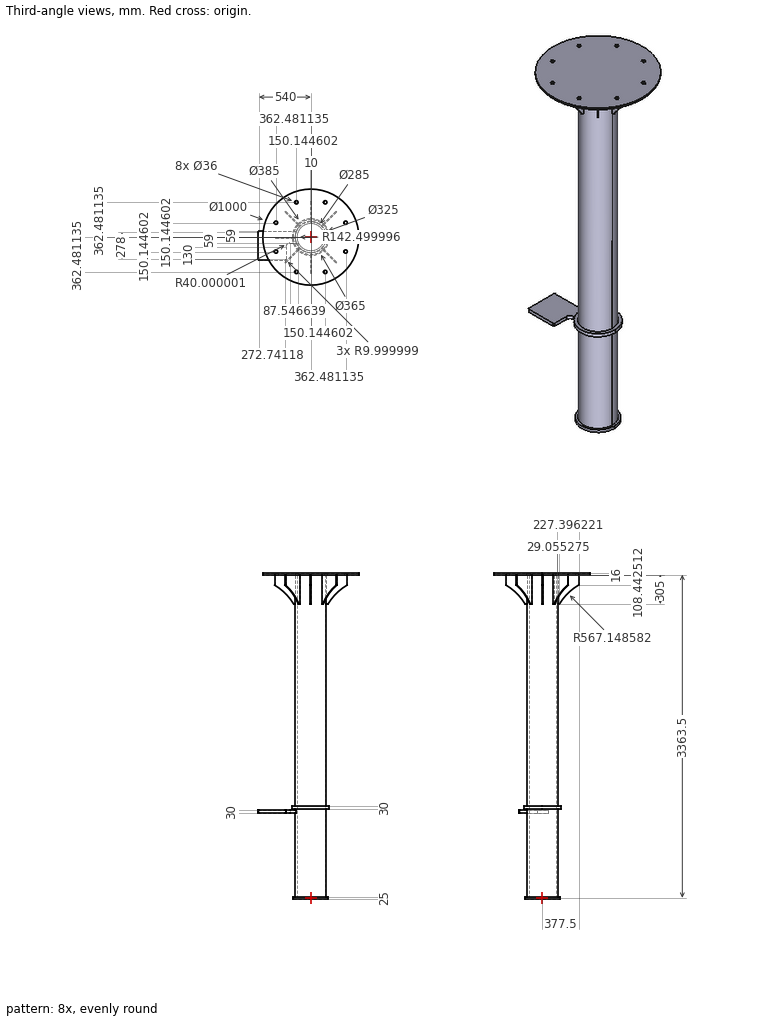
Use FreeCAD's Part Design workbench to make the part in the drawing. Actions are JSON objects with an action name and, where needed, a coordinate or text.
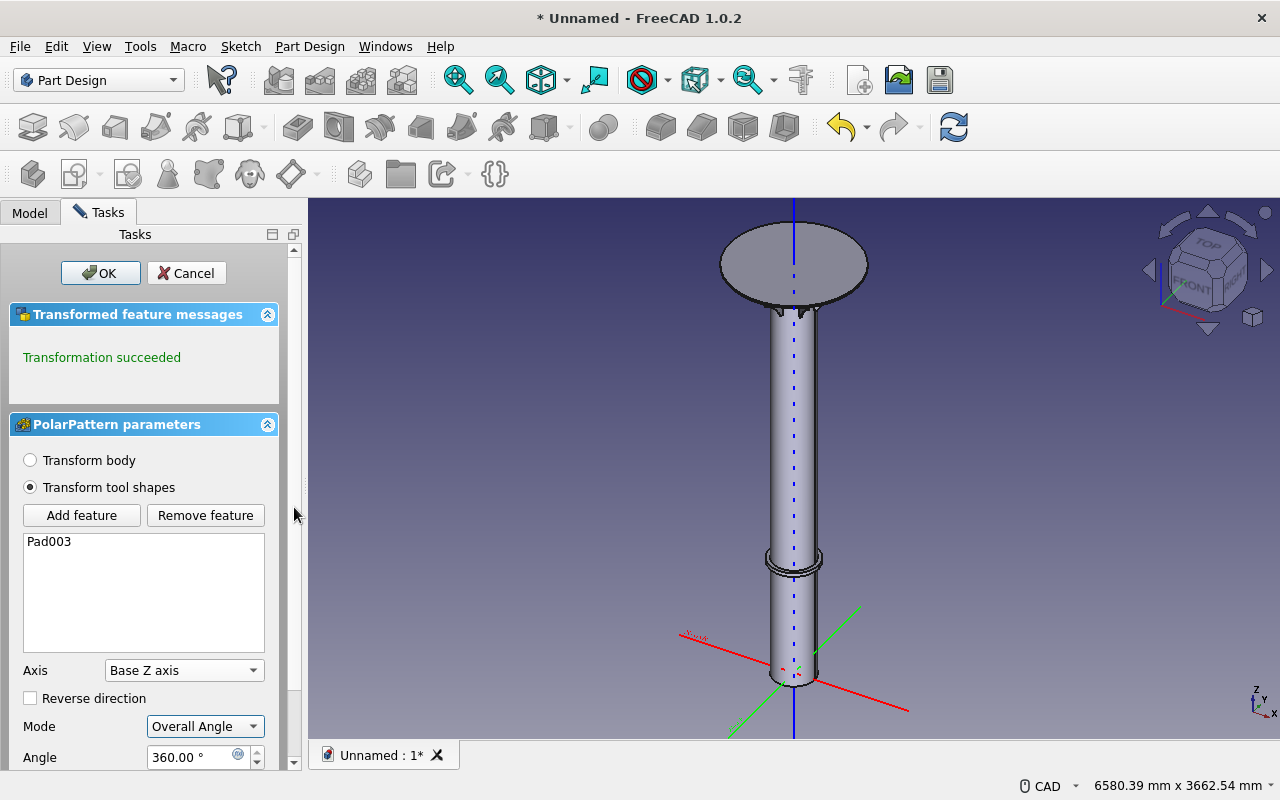
{"action": "left_click", "coordinate": [101, 273]}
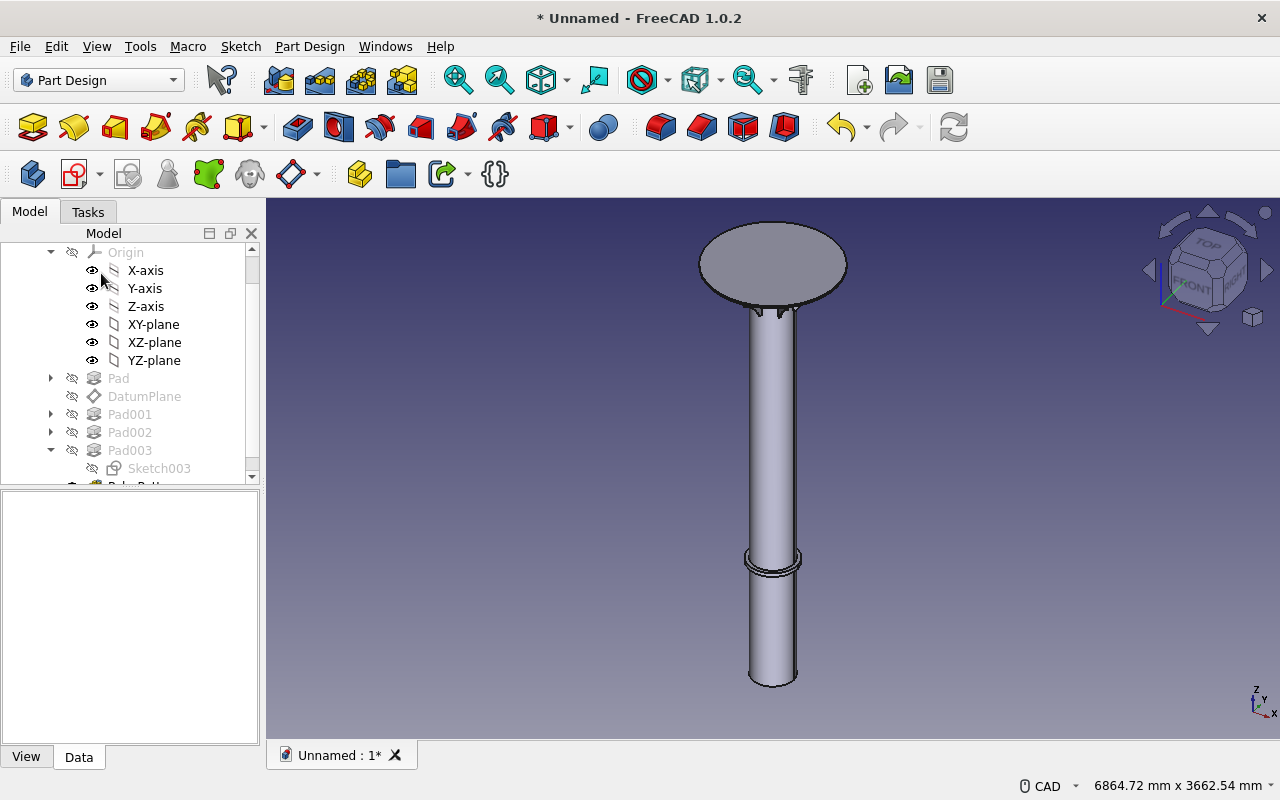
{"action": "key", "text": "5"}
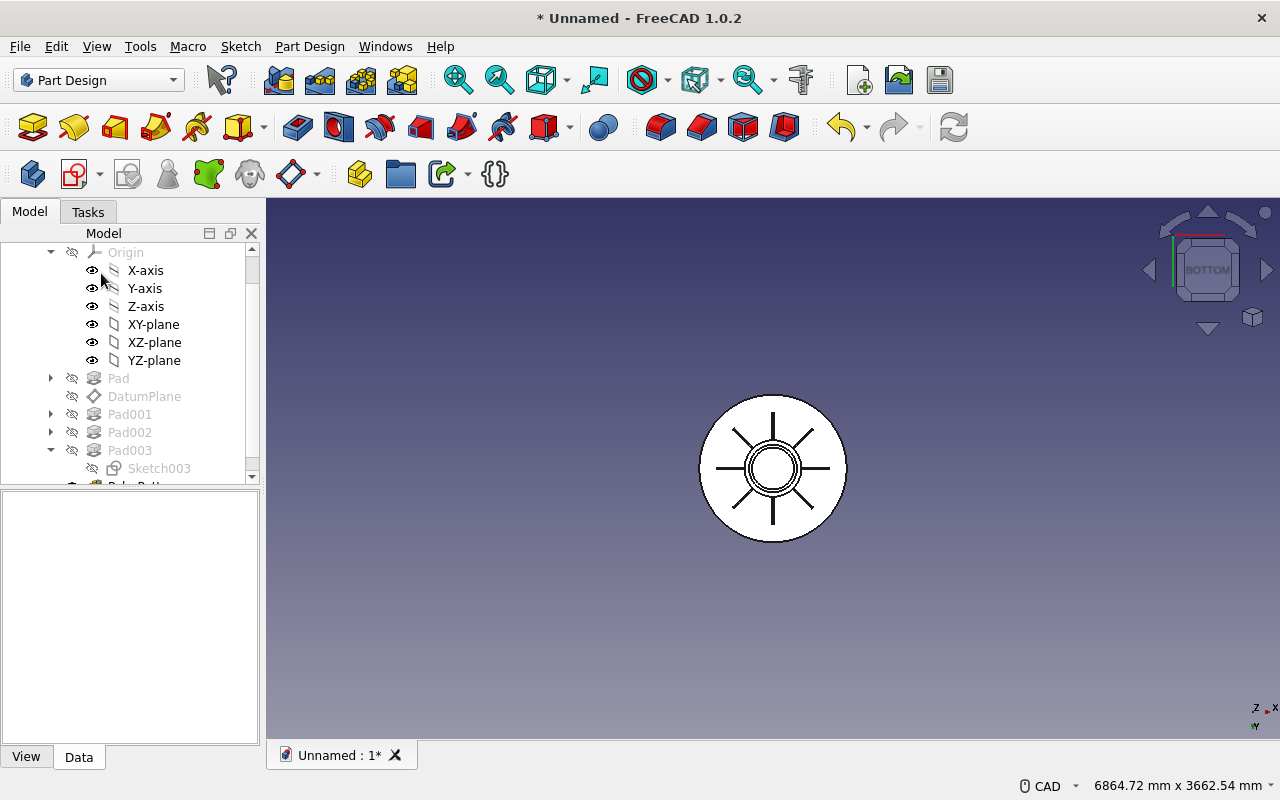
{"action": "left_click", "coordinate": [459, 80]}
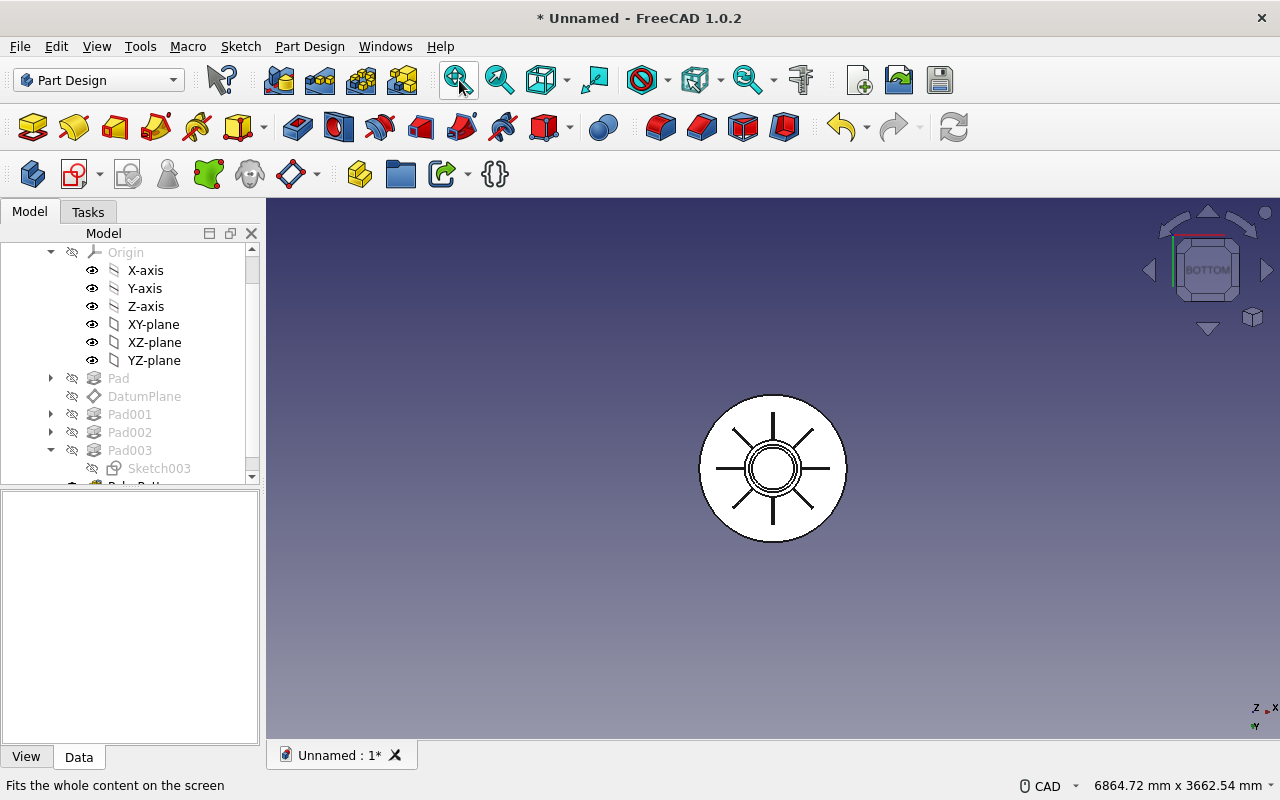
{"action": "left_click", "coordinate": [794, 425]}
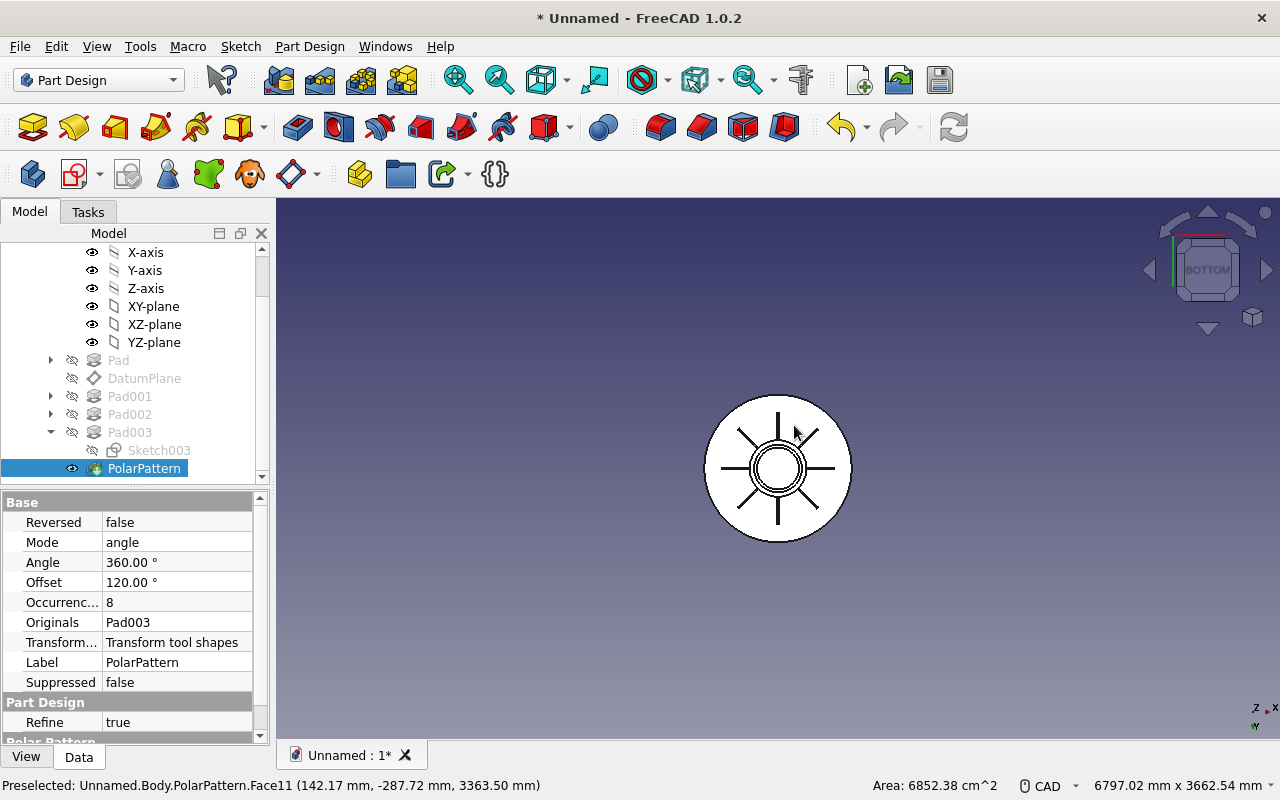
{"action": "left_click", "coordinate": [74, 174]}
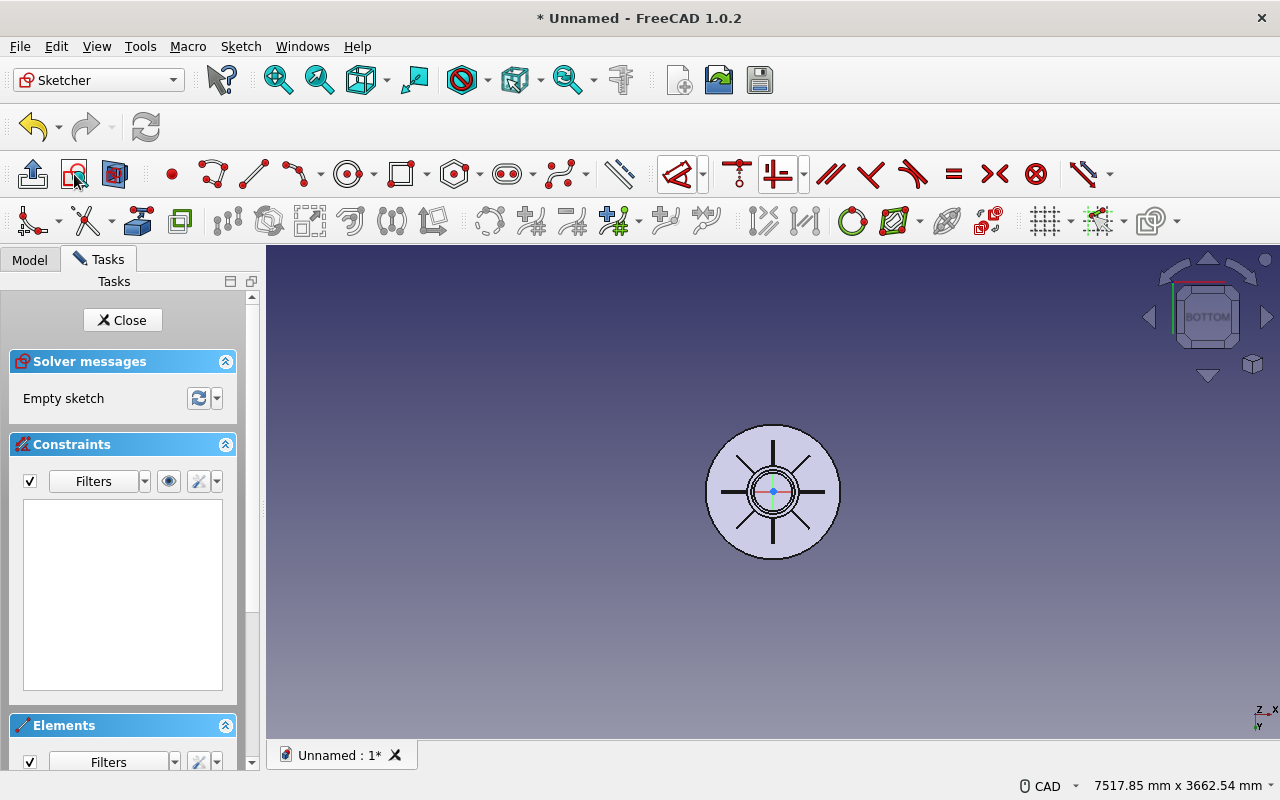
{"action": "scroll", "coordinate": [803, 492], "scroll_direction": "up", "scroll_amount": 6}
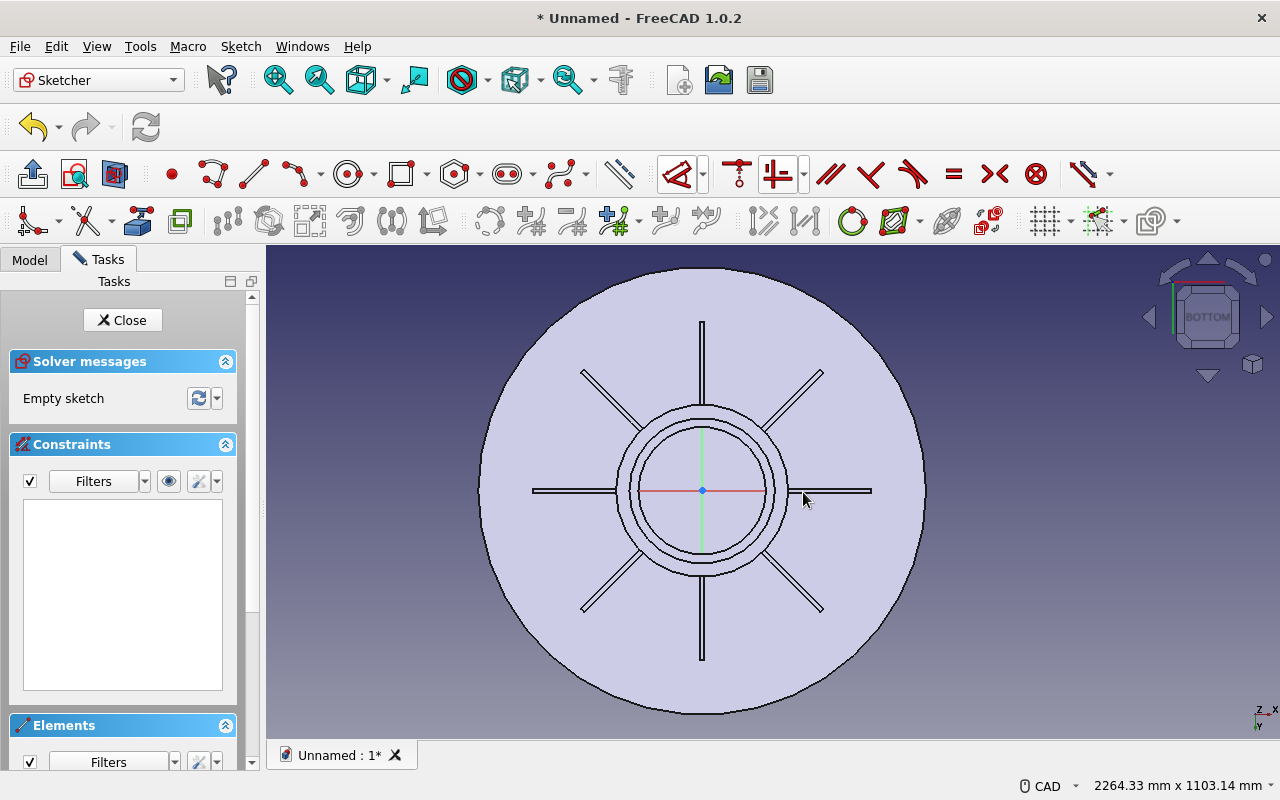
{"action": "key", "text": "g c"}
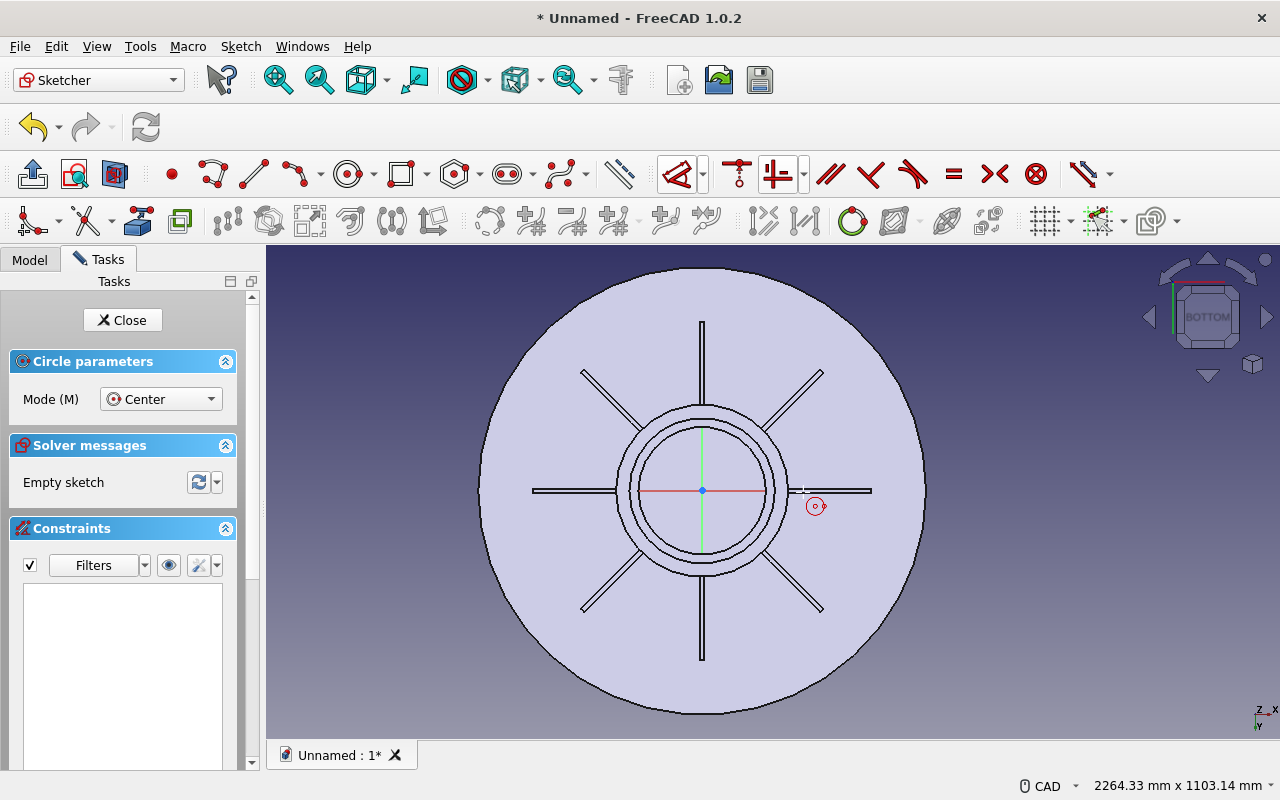
{"action": "scroll", "coordinate": [635, 653], "scroll_direction": "up", "scroll_amount": 6}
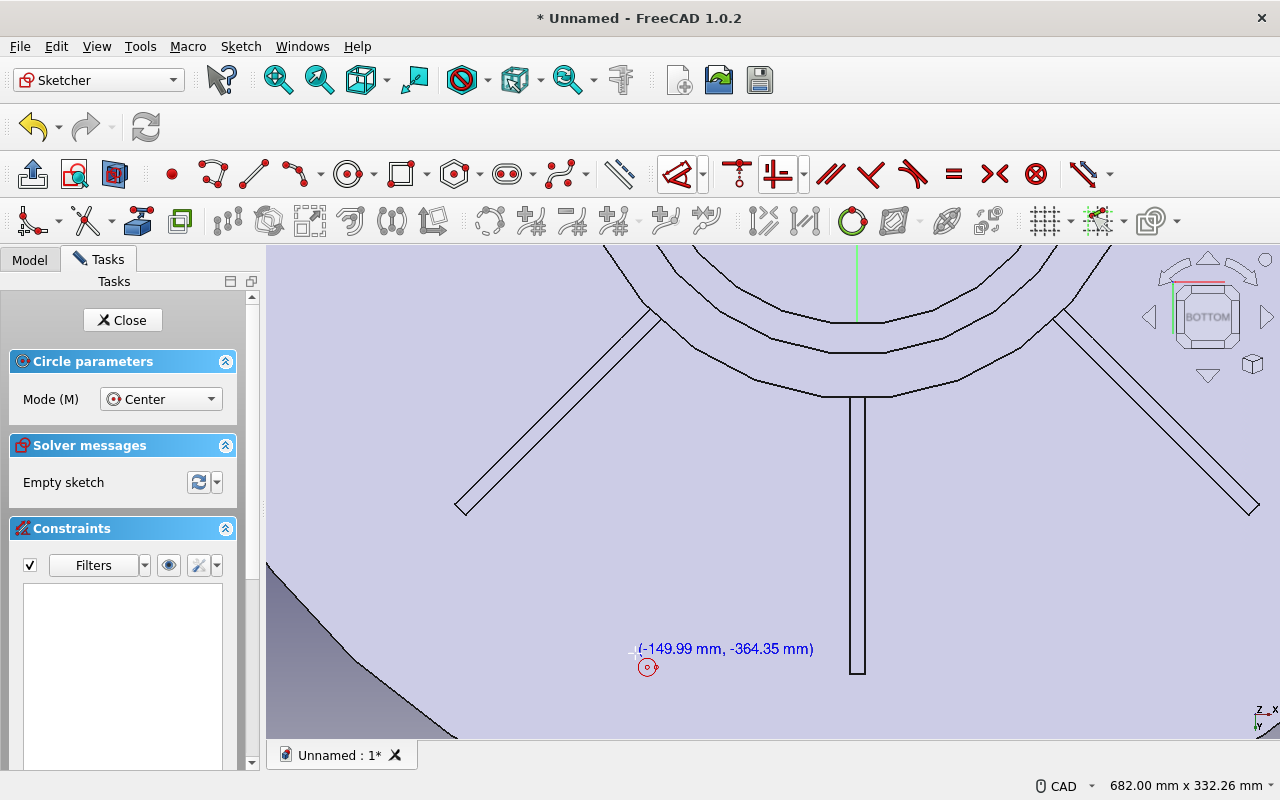
{"action": "left_click", "coordinate": [634, 652]}
{"action": "left_click", "coordinate": [653, 633]}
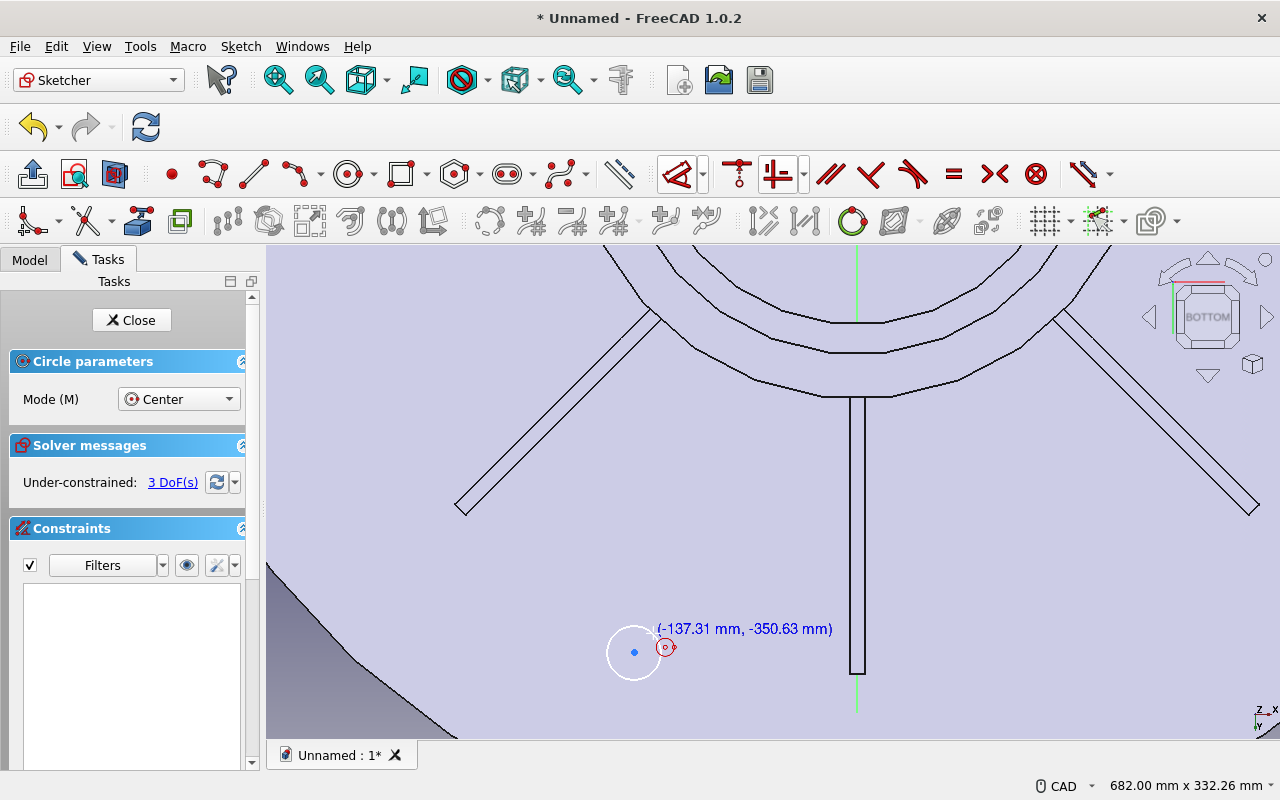
{"action": "left_click", "coordinate": [318, 336]}
{"action": "left_click", "coordinate": [337, 317]}